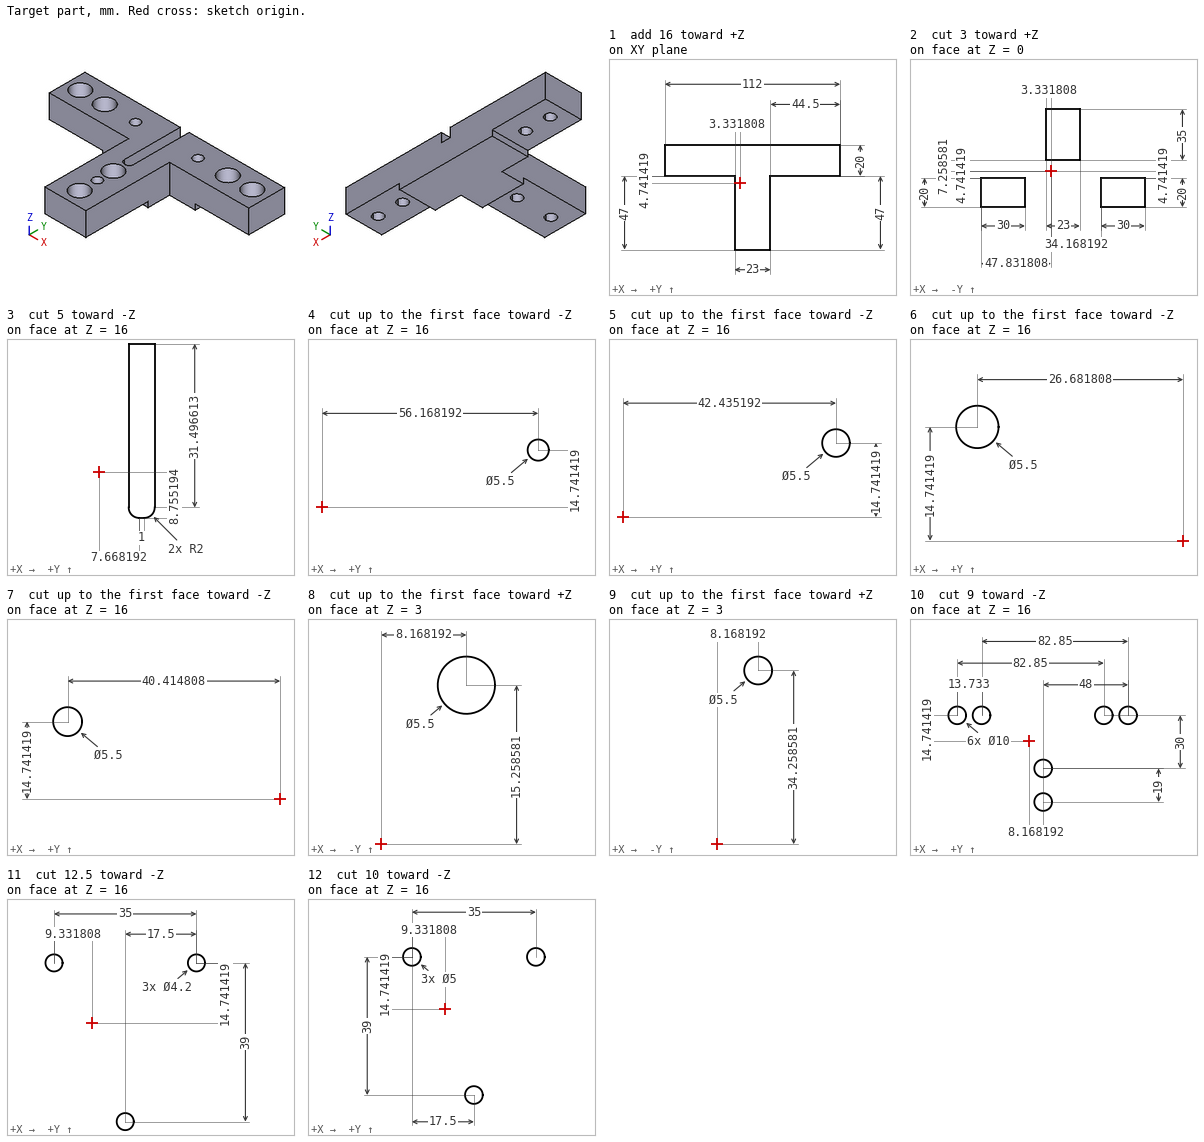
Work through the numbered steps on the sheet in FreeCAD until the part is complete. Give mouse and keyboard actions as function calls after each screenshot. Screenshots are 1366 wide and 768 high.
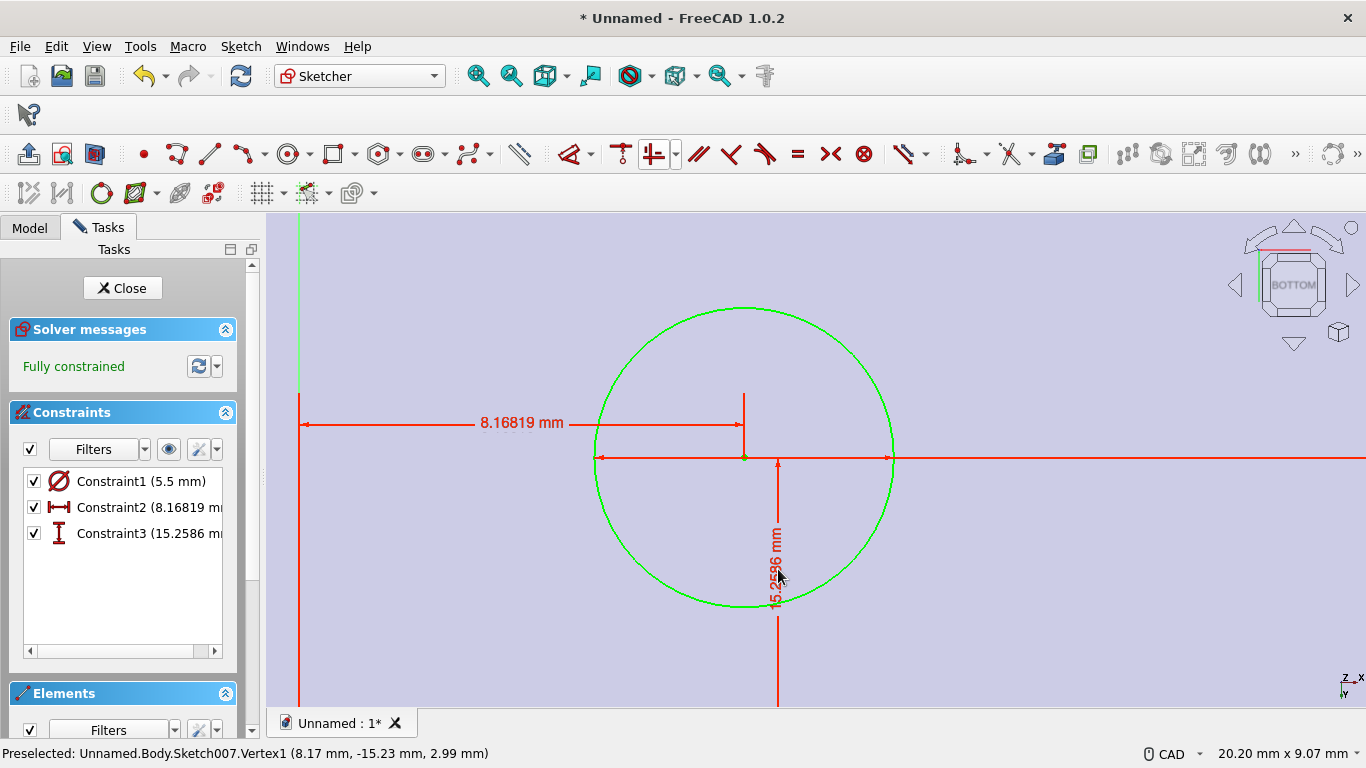
click(123, 288)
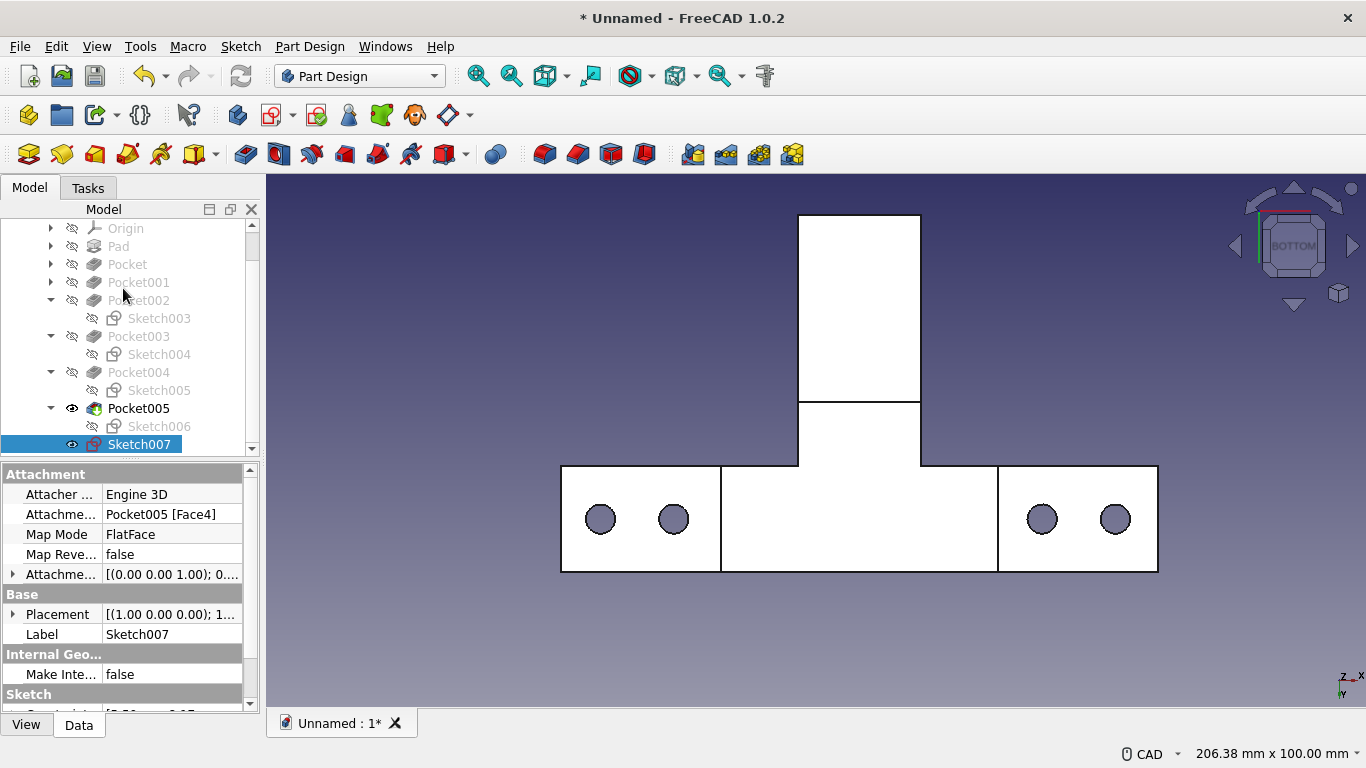
click(246, 154)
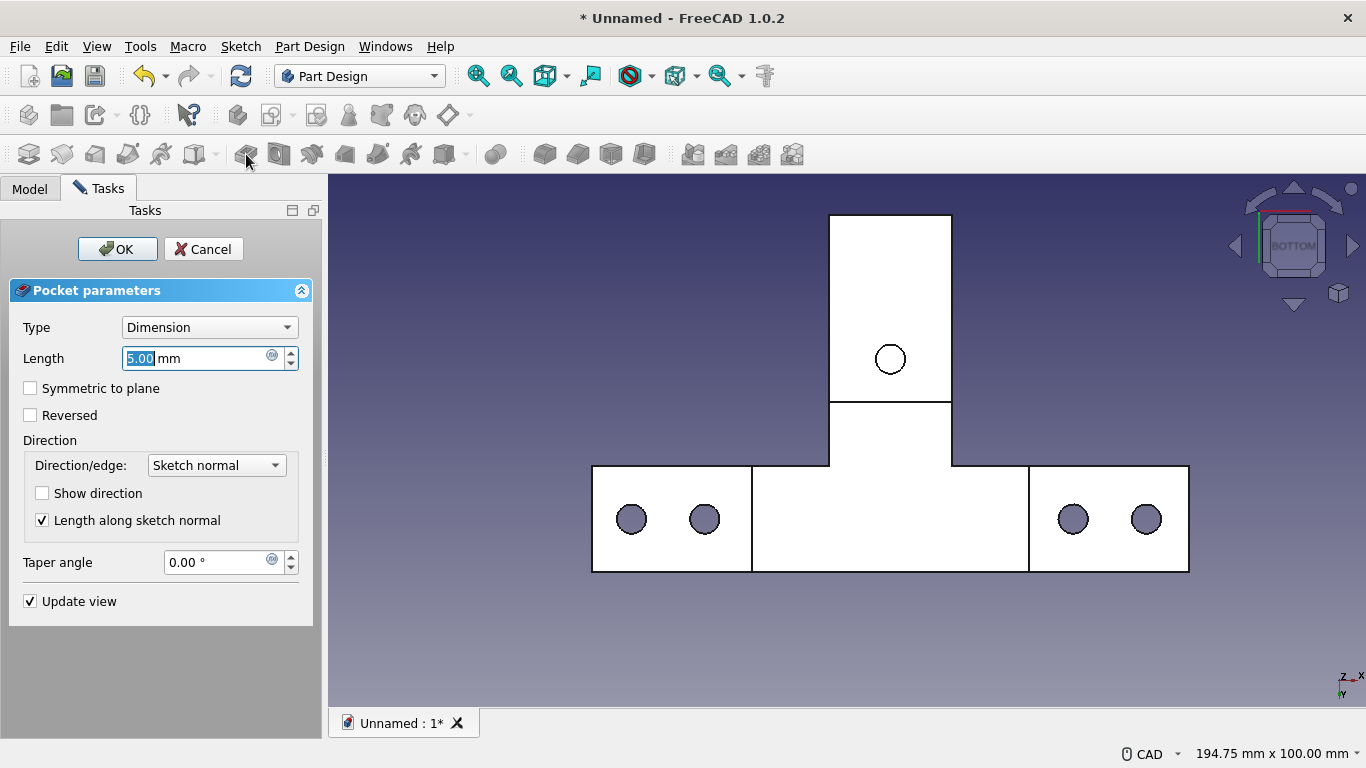
click(210, 328)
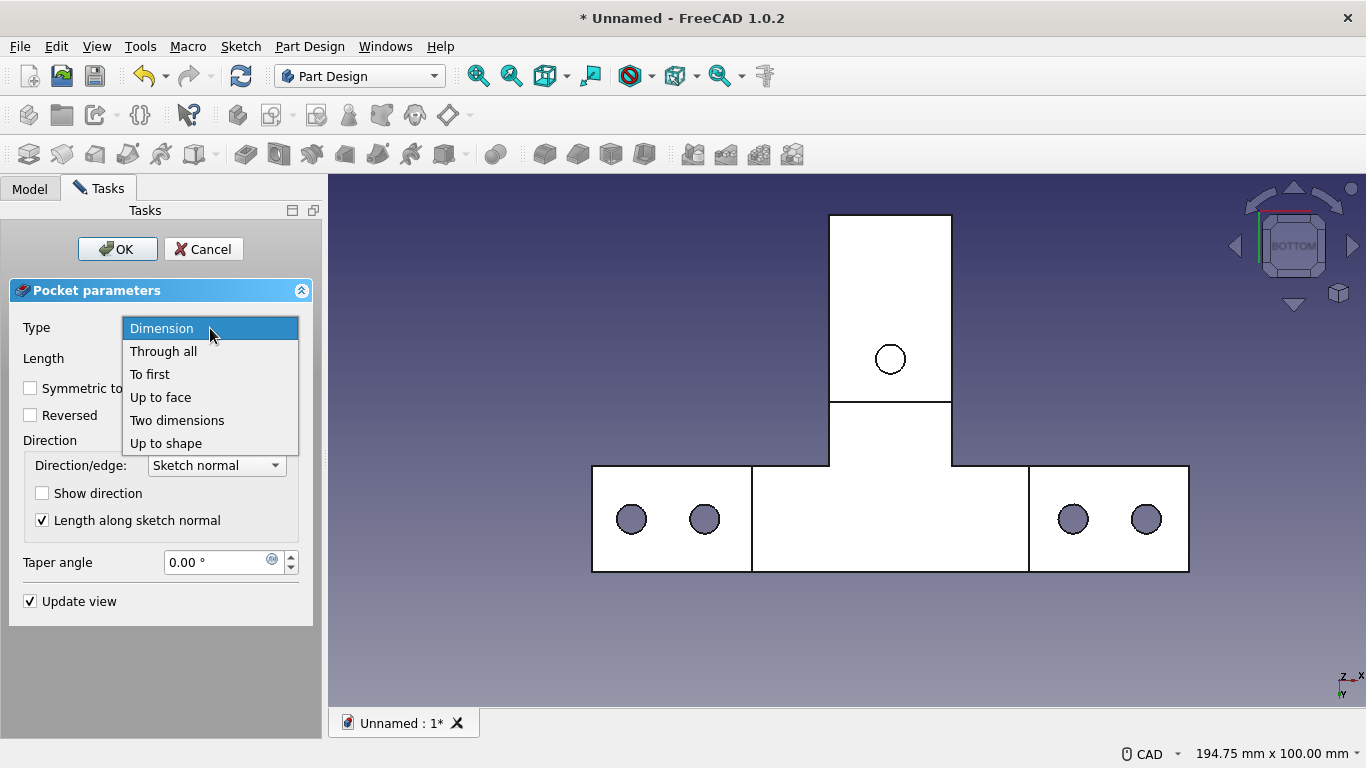
click(208, 374)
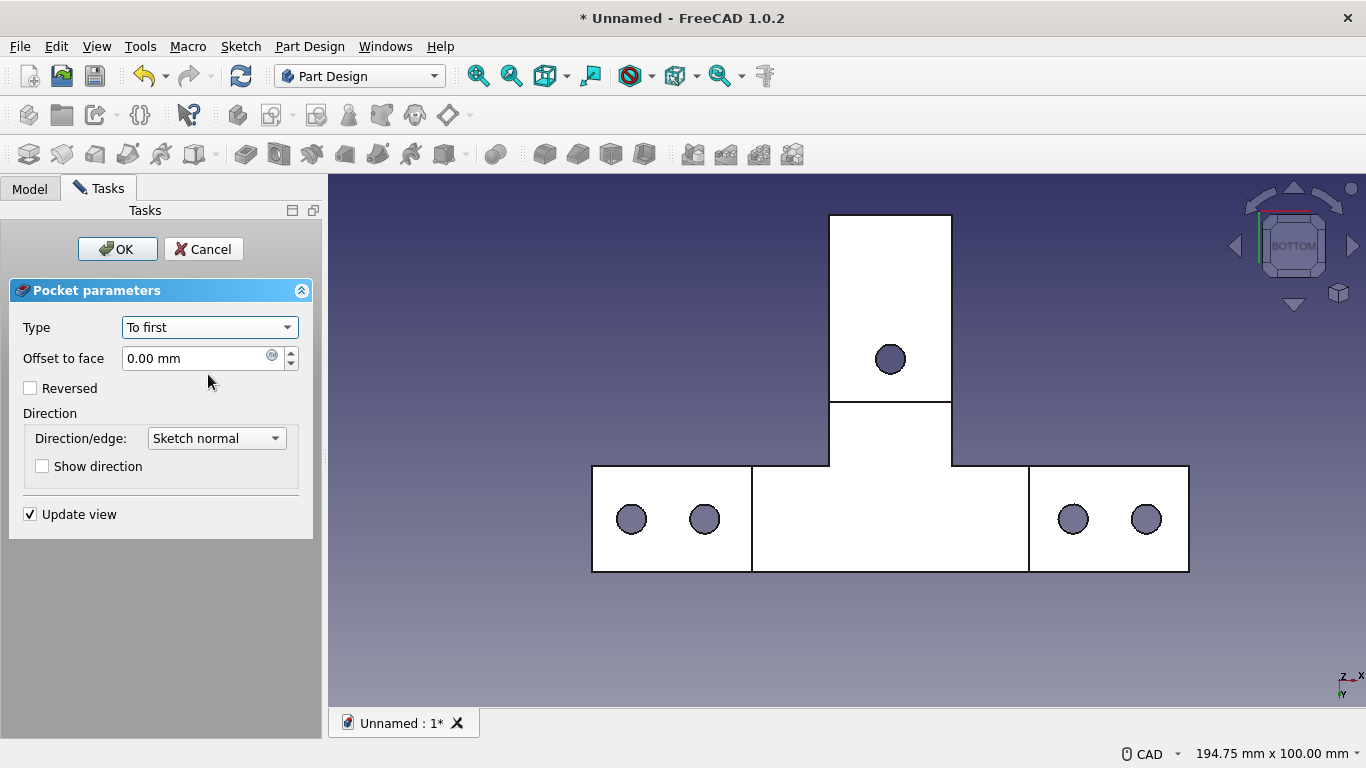
click(118, 249)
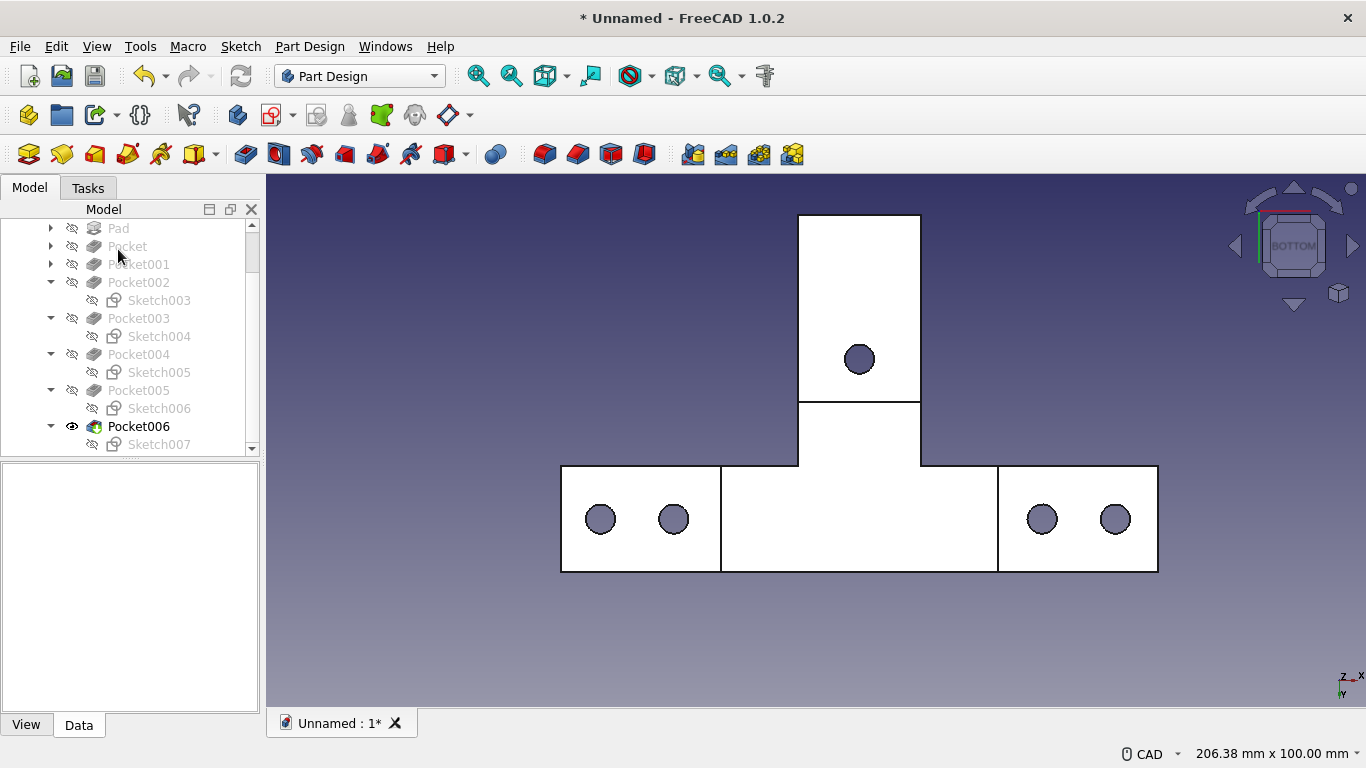
click(860, 281)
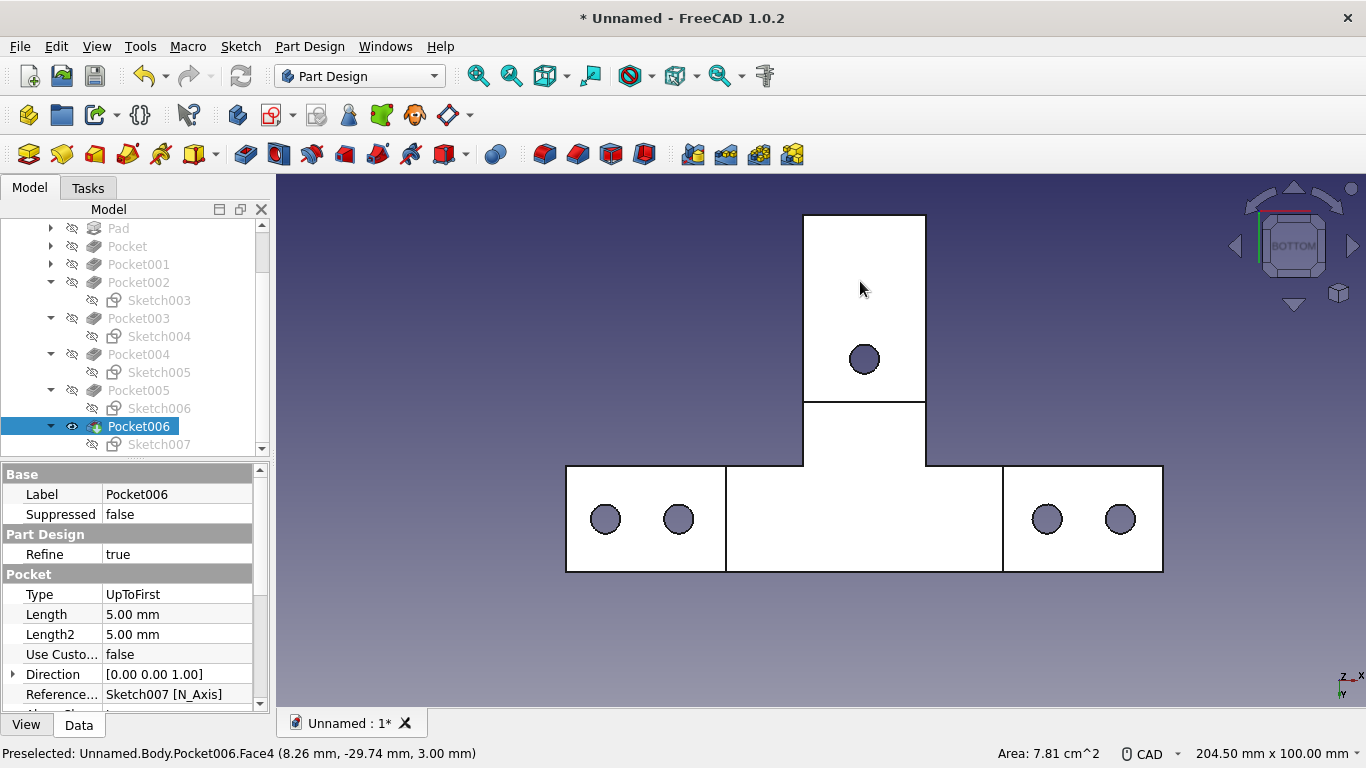
click(270, 116)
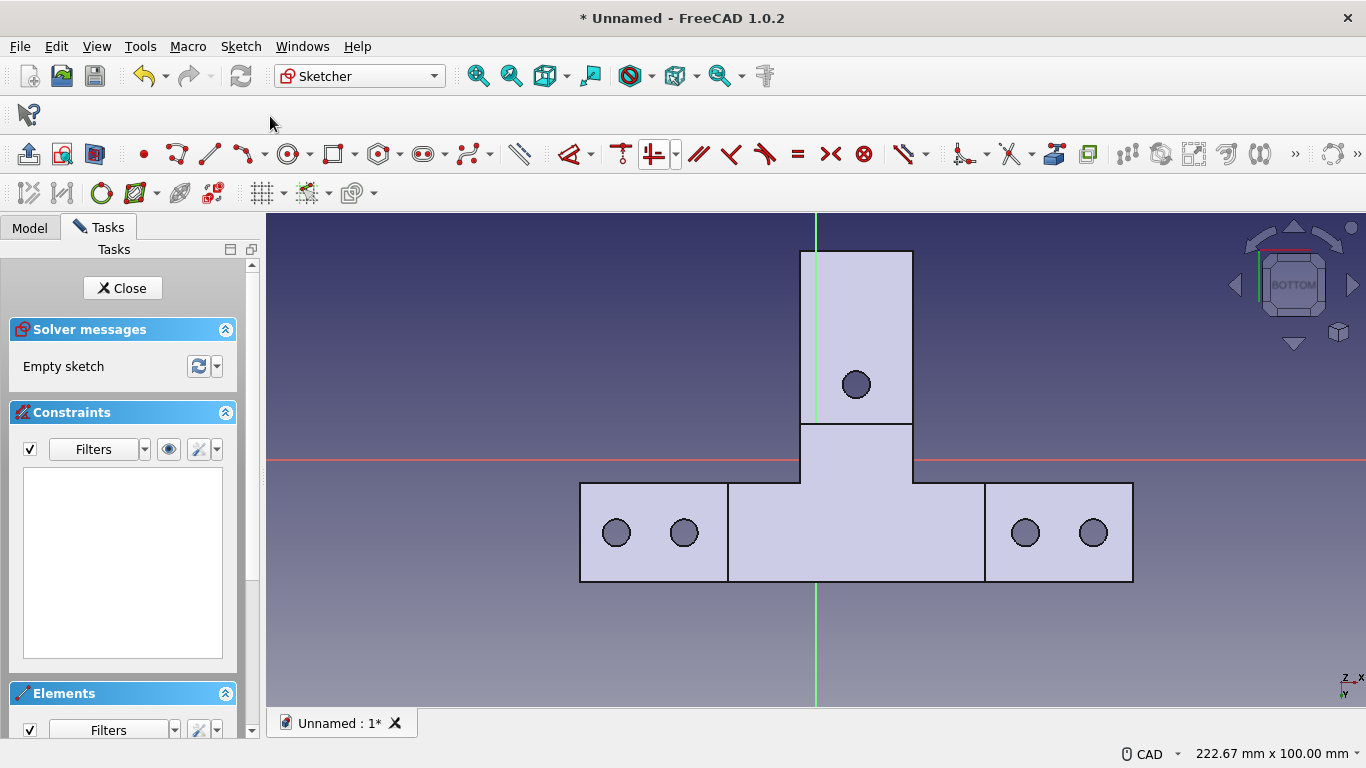
scroll(867, 274, up, 12)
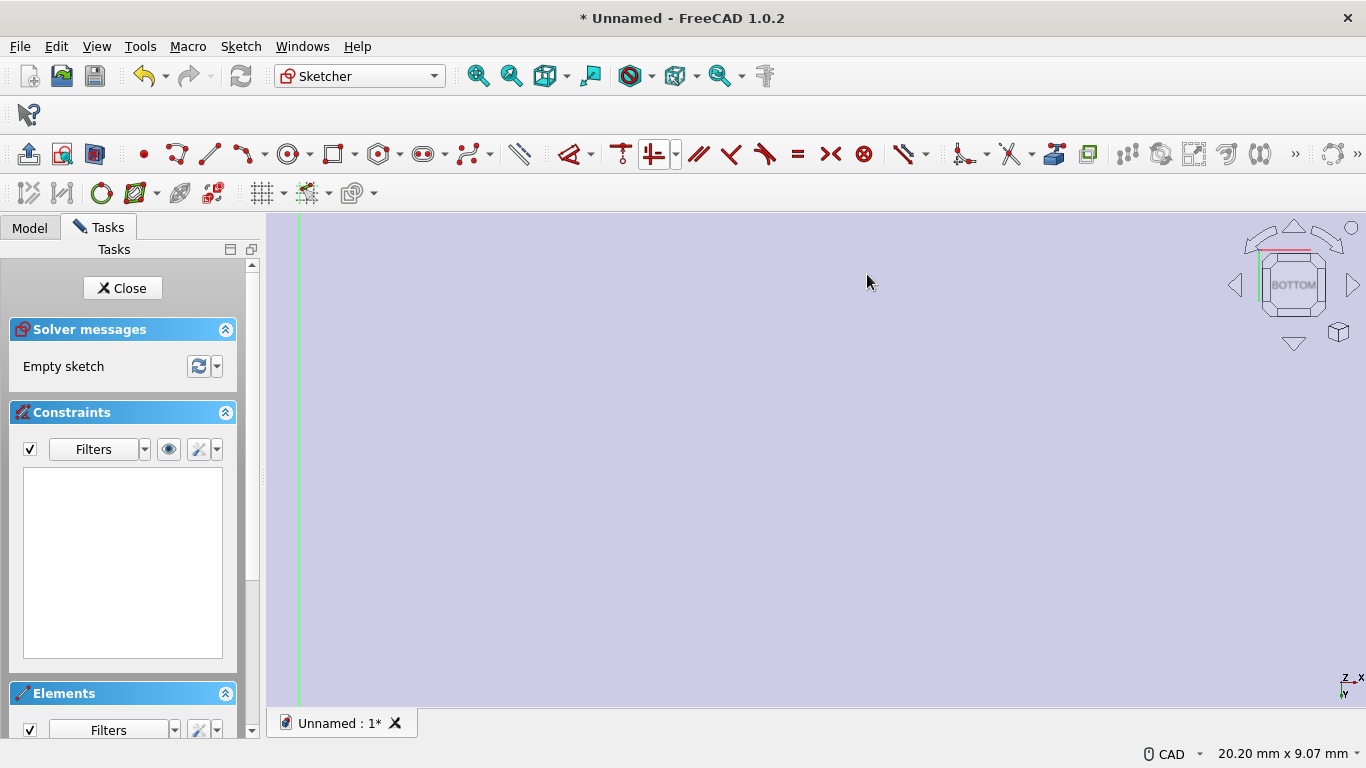
click(288, 154)